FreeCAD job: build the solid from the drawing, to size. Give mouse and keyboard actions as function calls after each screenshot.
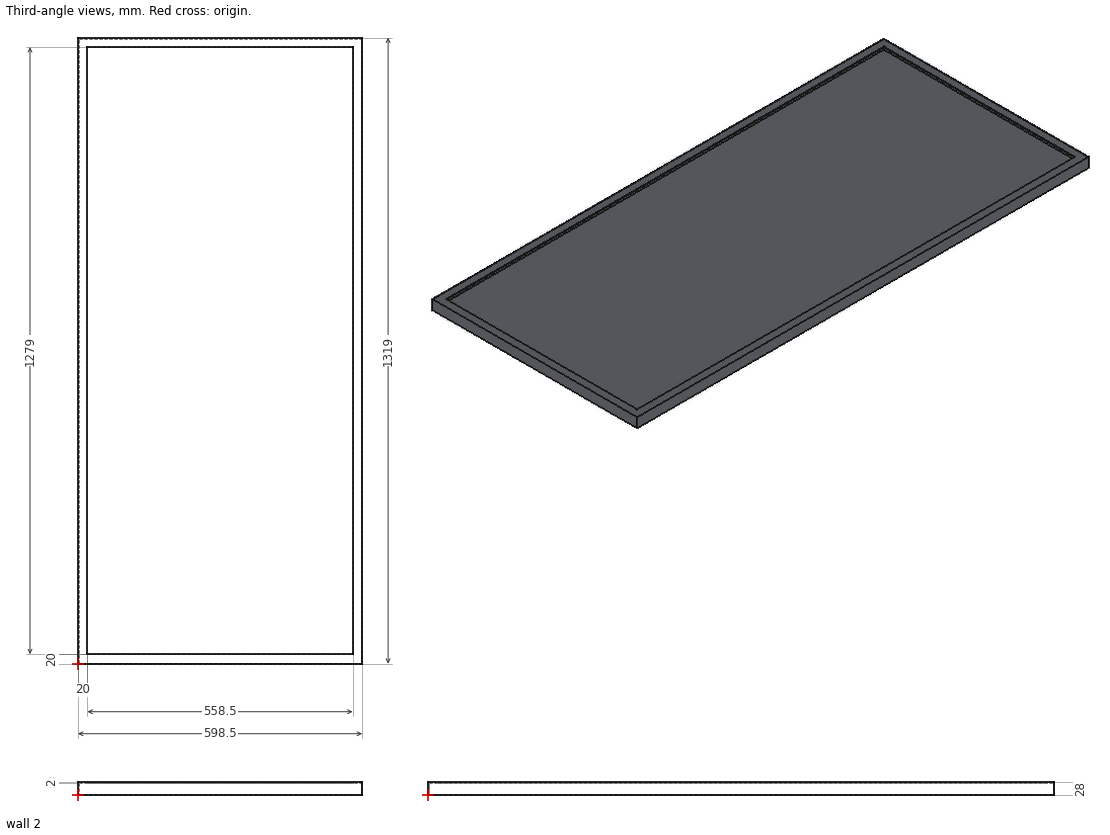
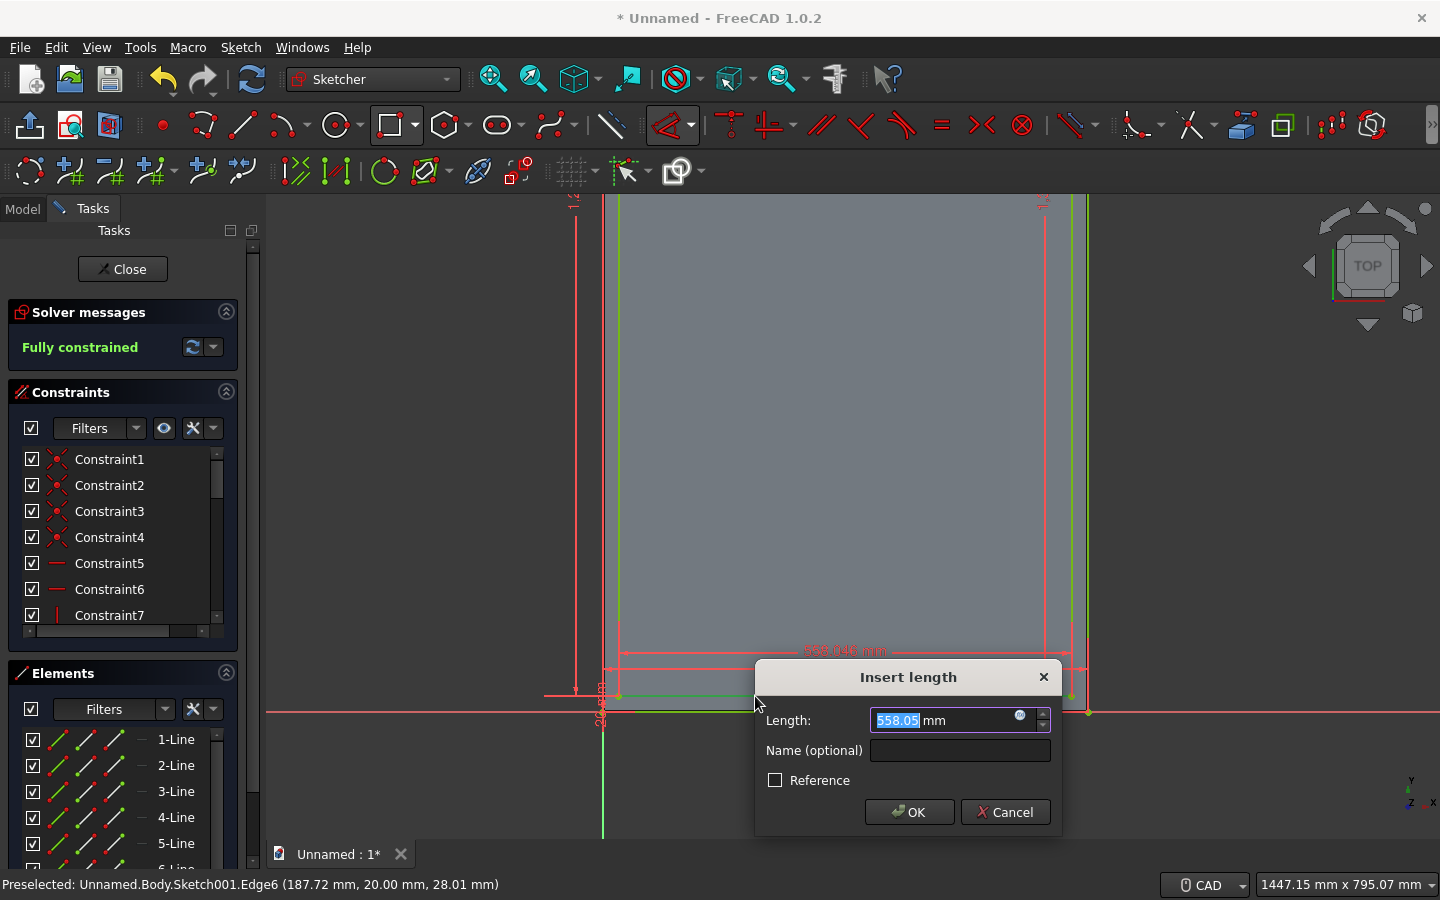
text(558.5)
key(Return)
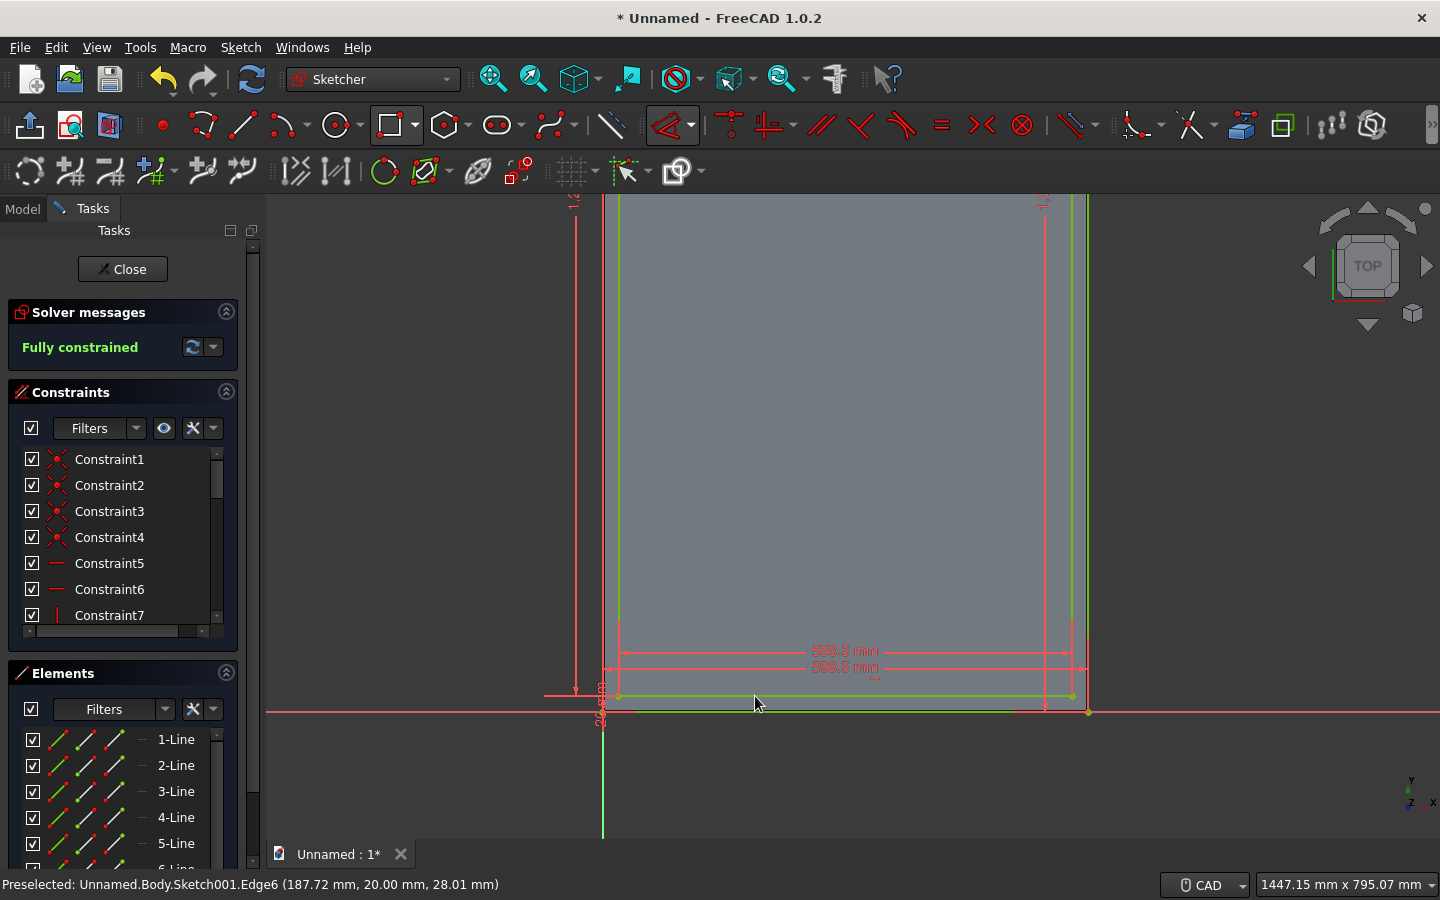
click(123, 269)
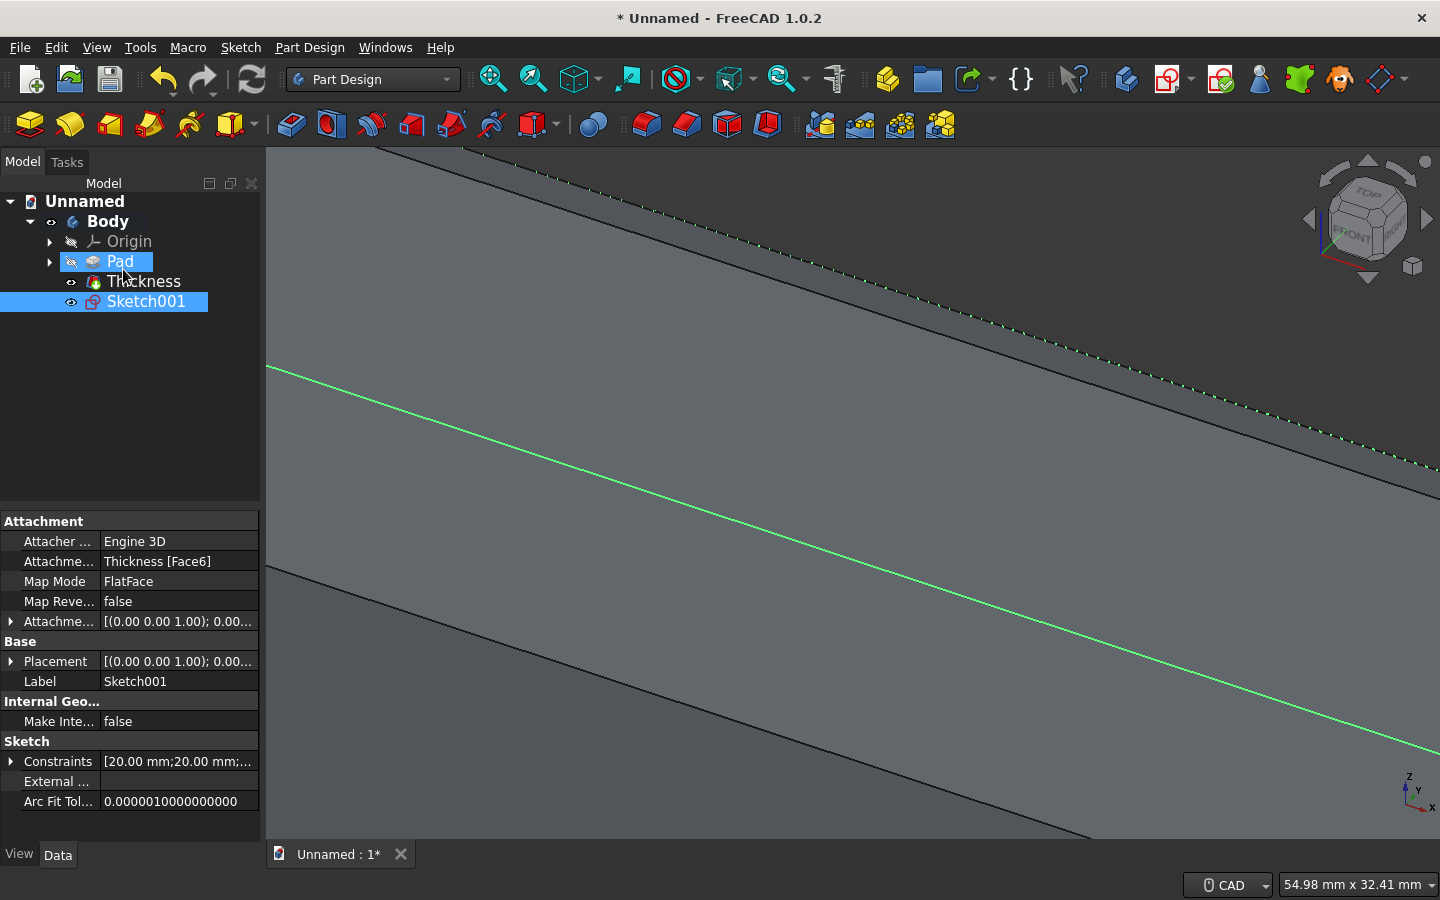
click(30, 124)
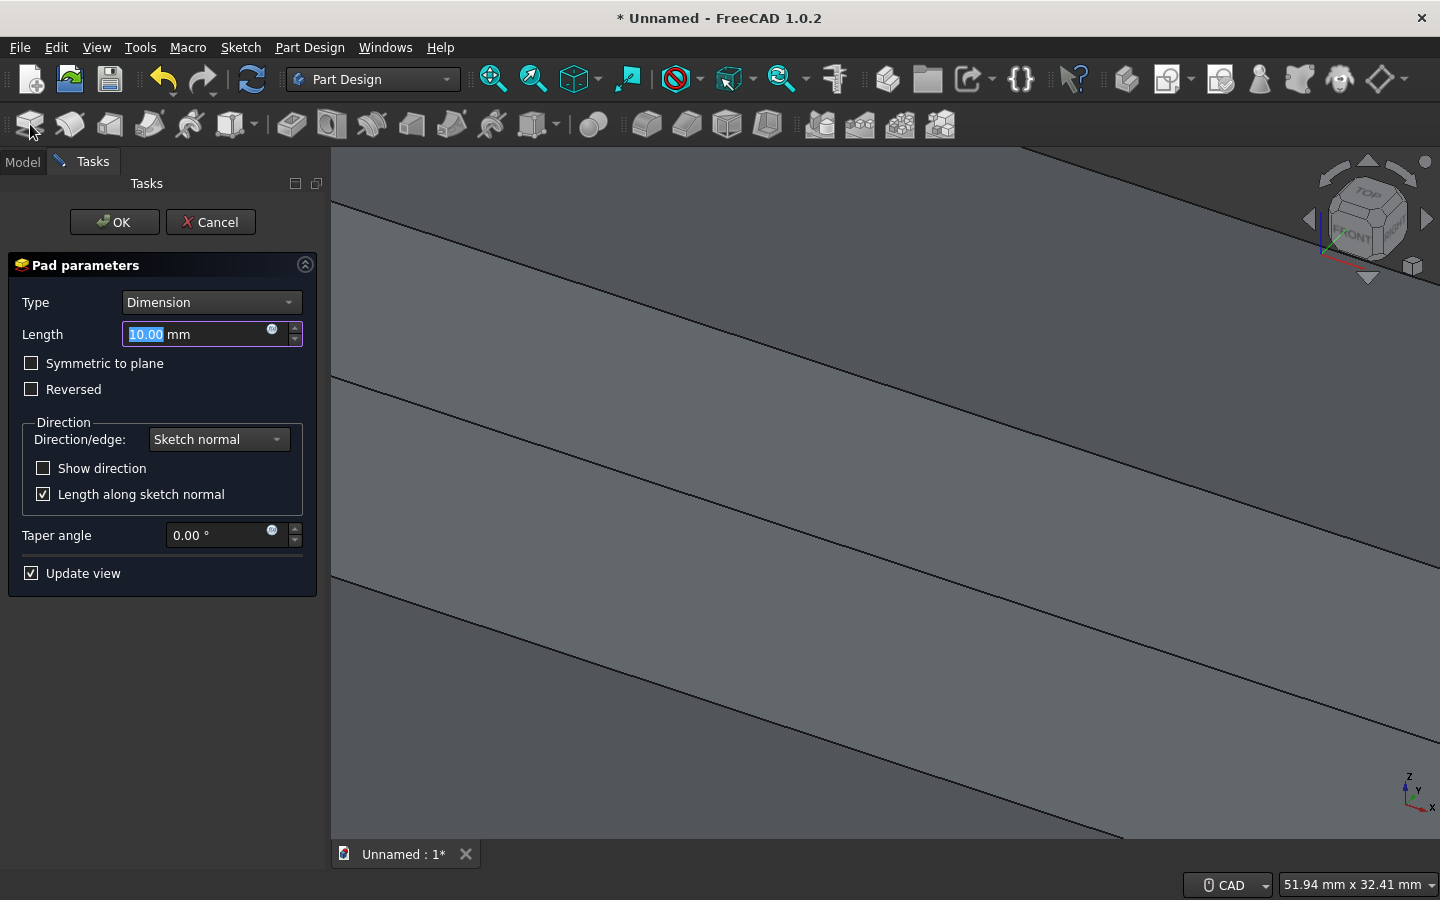
text(2)
key(Tab)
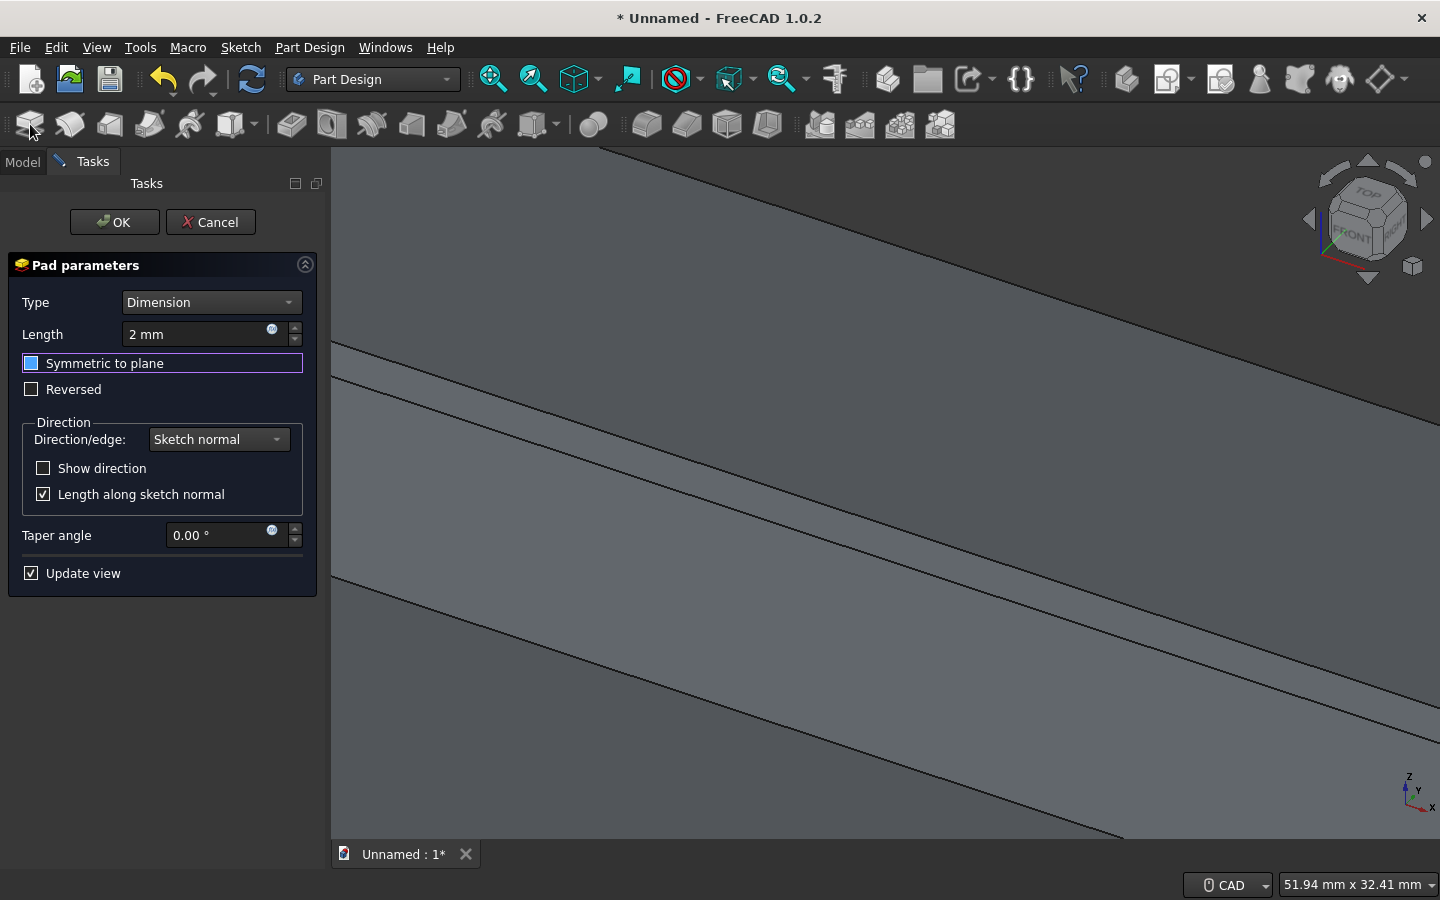
click(30, 389)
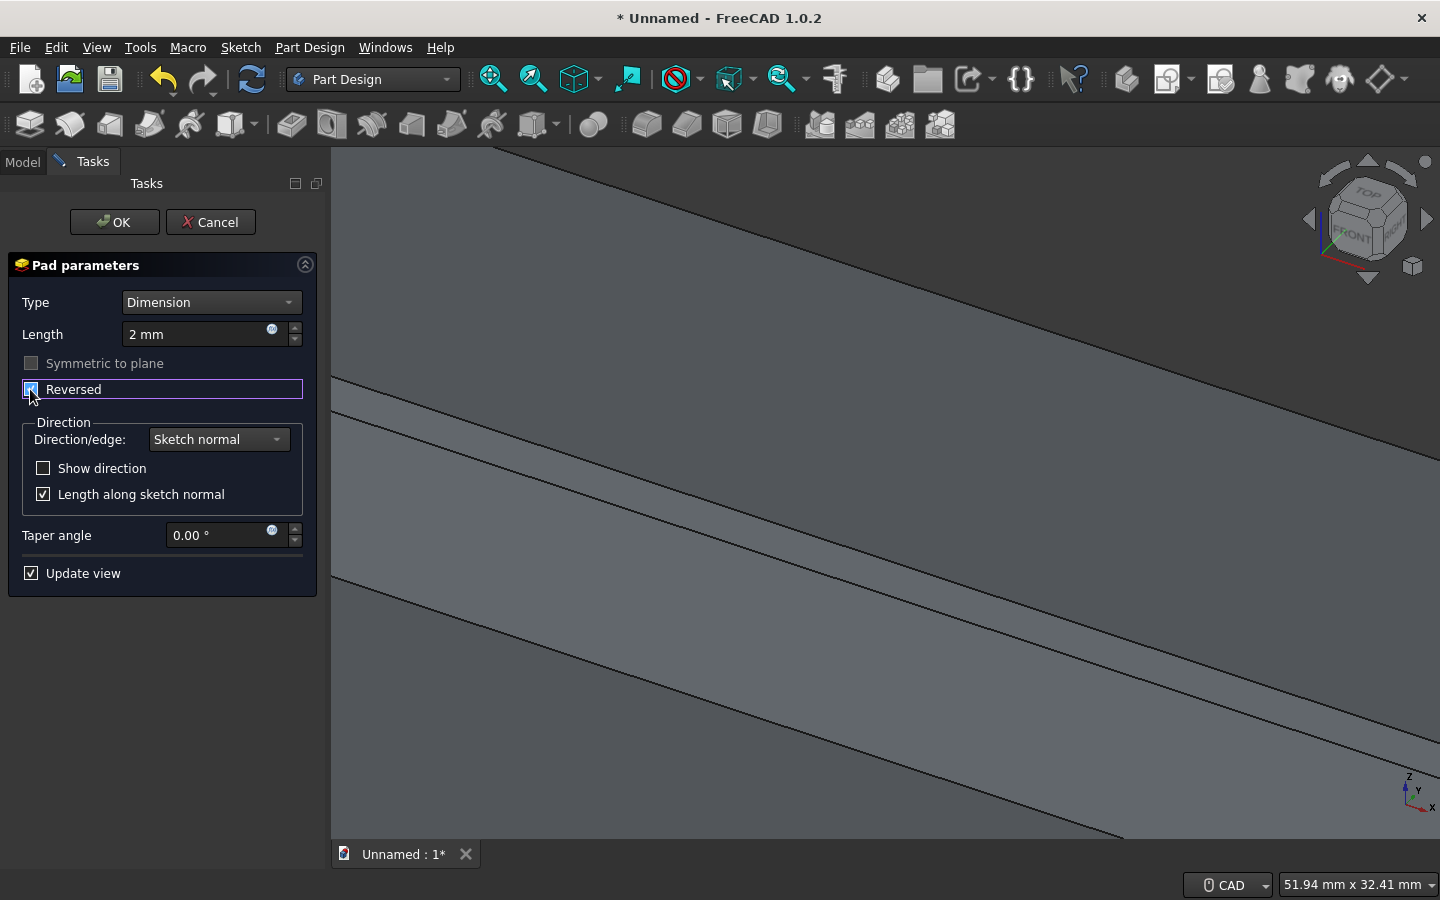
click(115, 222)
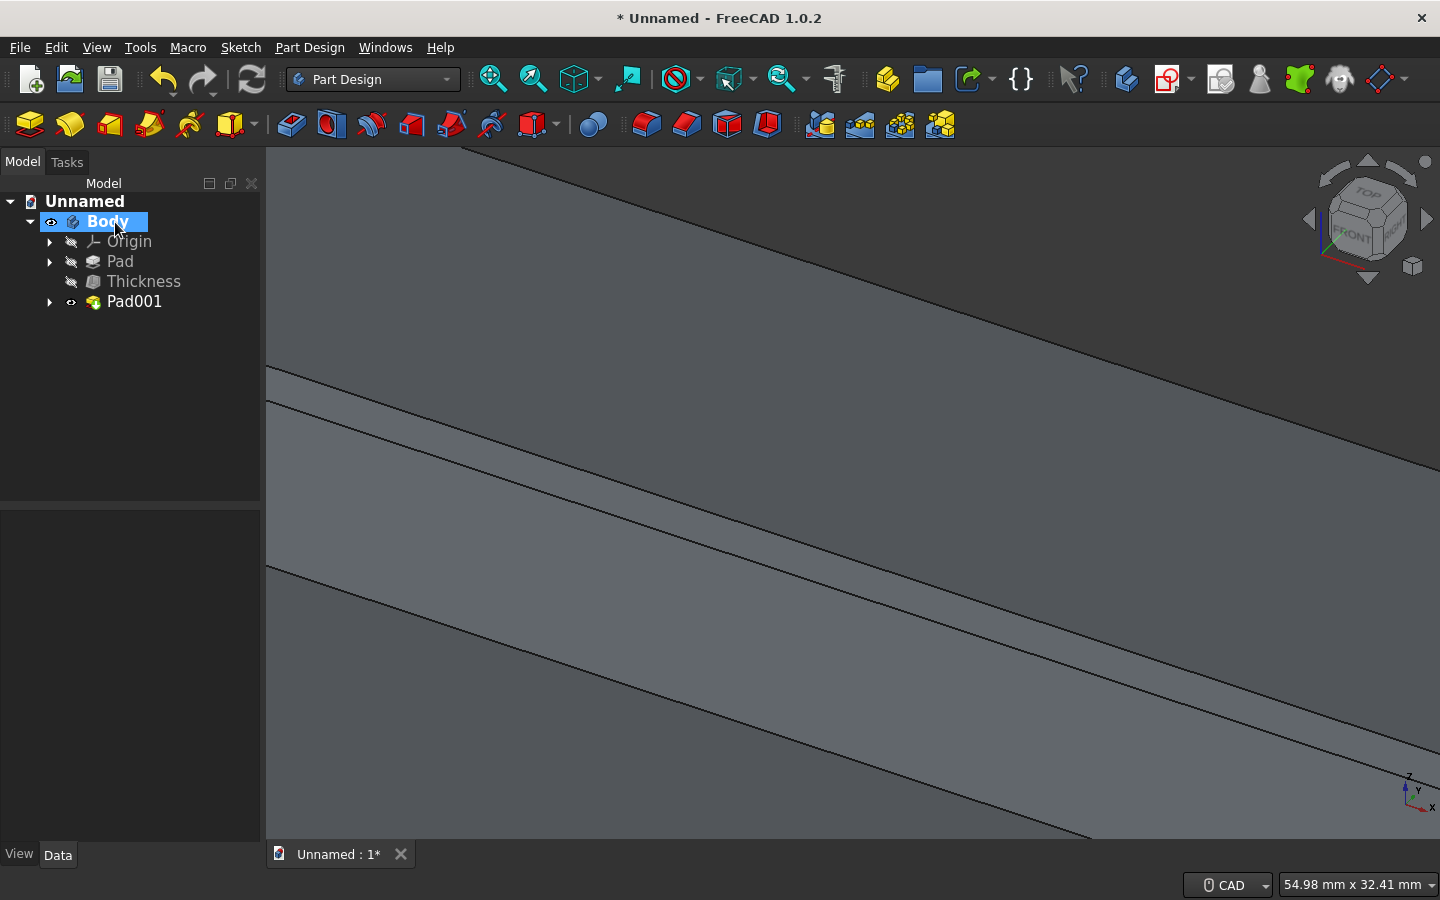
key(0)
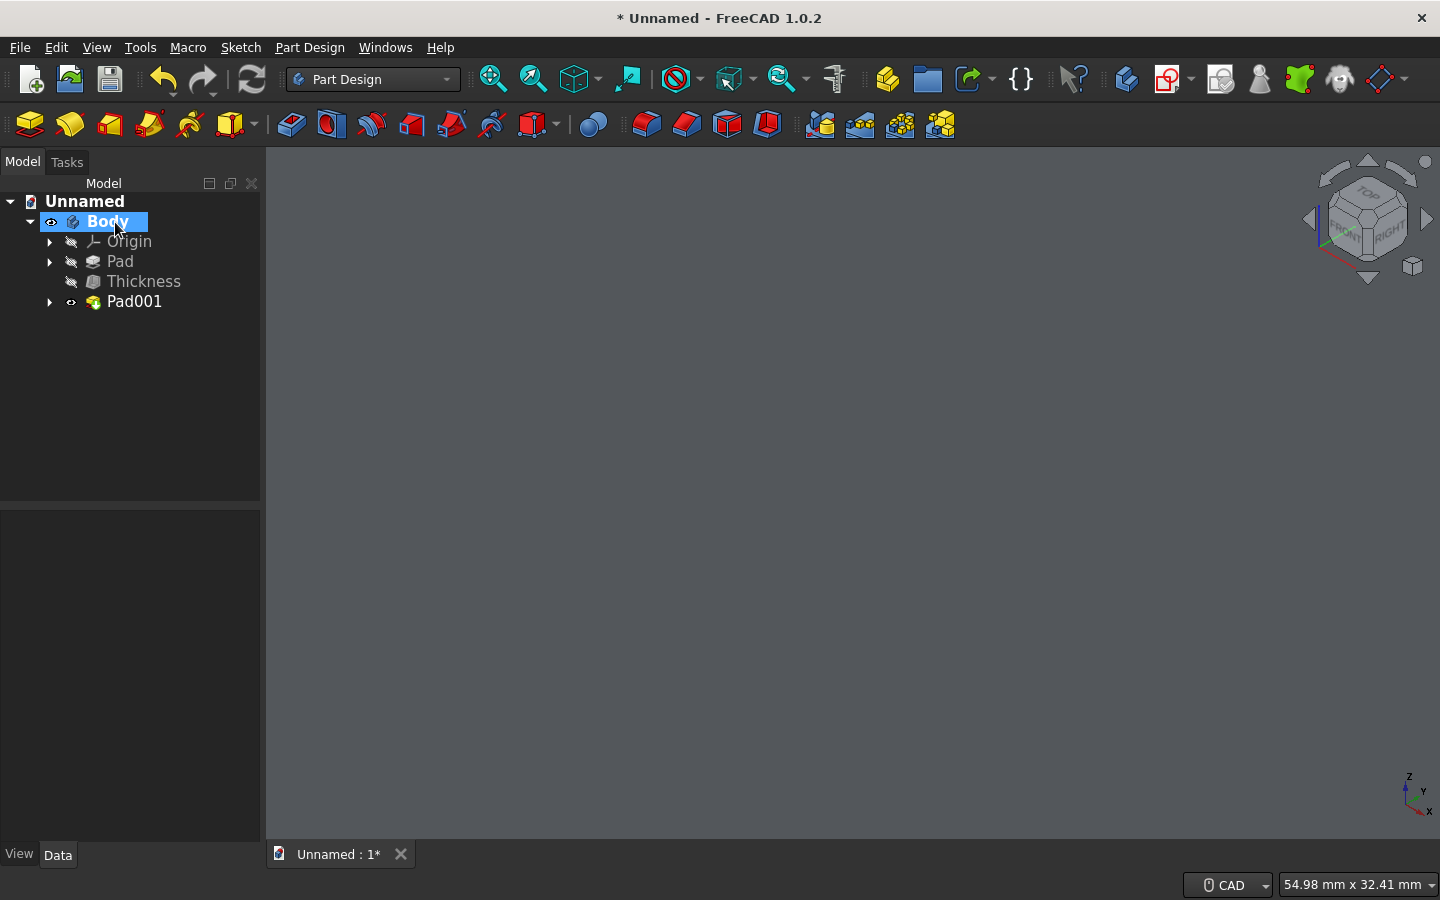
click(494, 80)